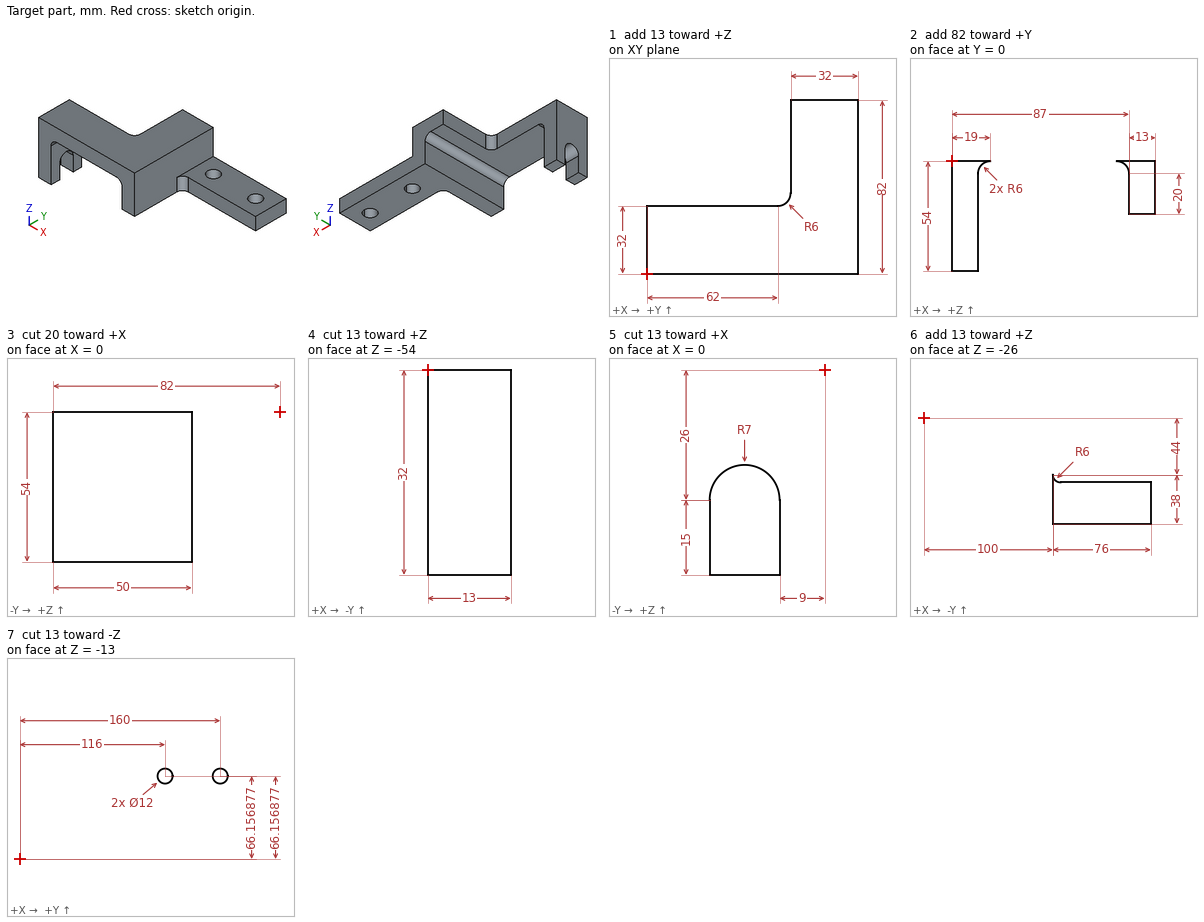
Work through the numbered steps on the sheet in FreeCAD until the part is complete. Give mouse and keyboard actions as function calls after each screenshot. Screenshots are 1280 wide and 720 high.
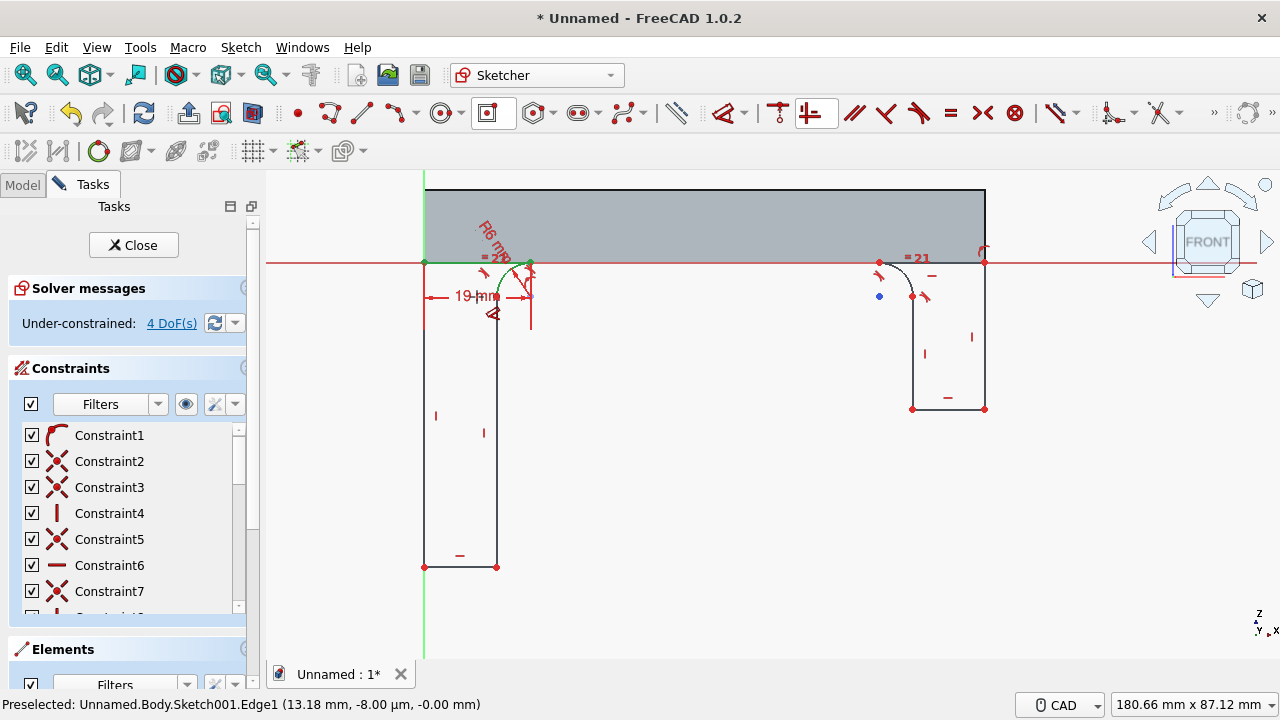
click(424, 354)
click(390, 415)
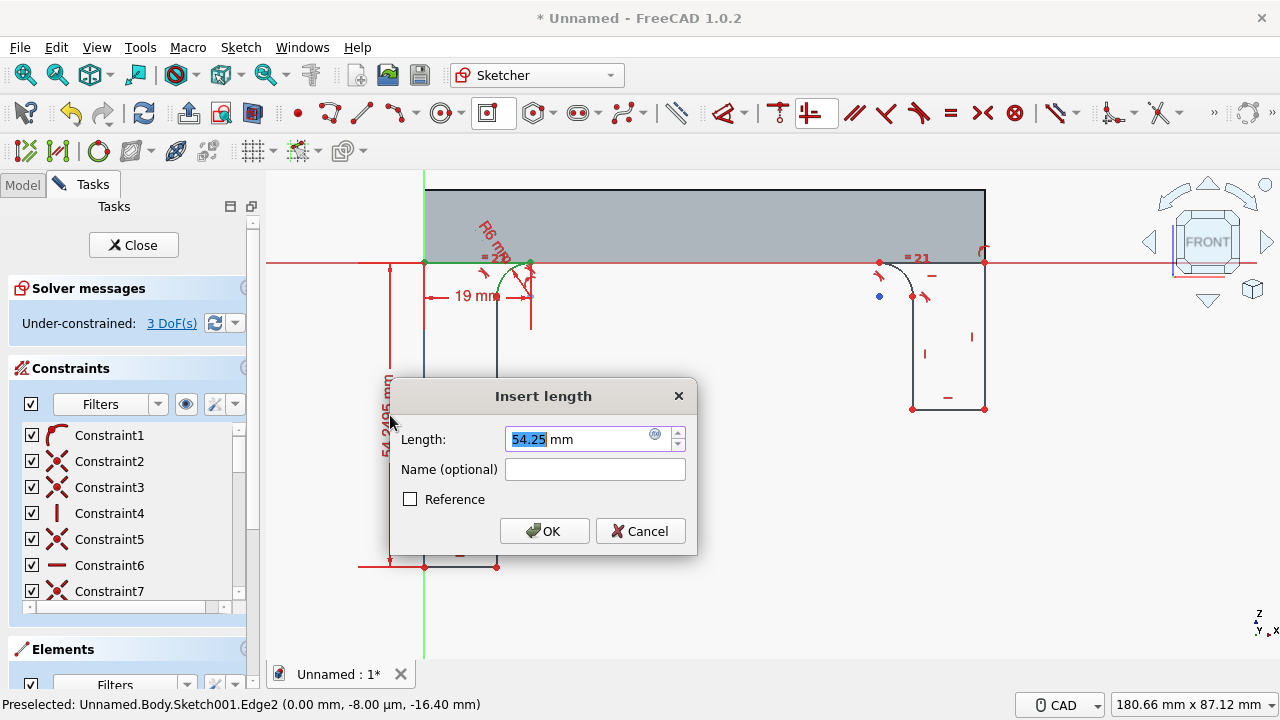
text(54)
key(Return)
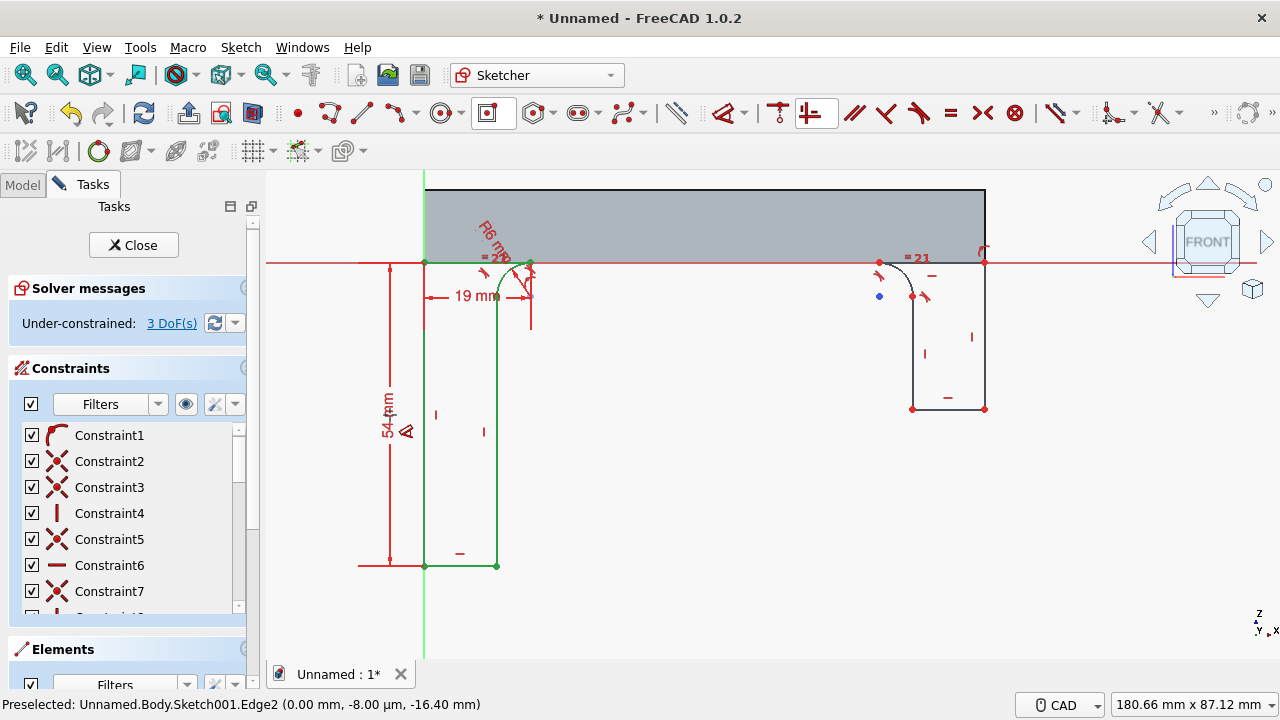
click(913, 331)
click(947, 353)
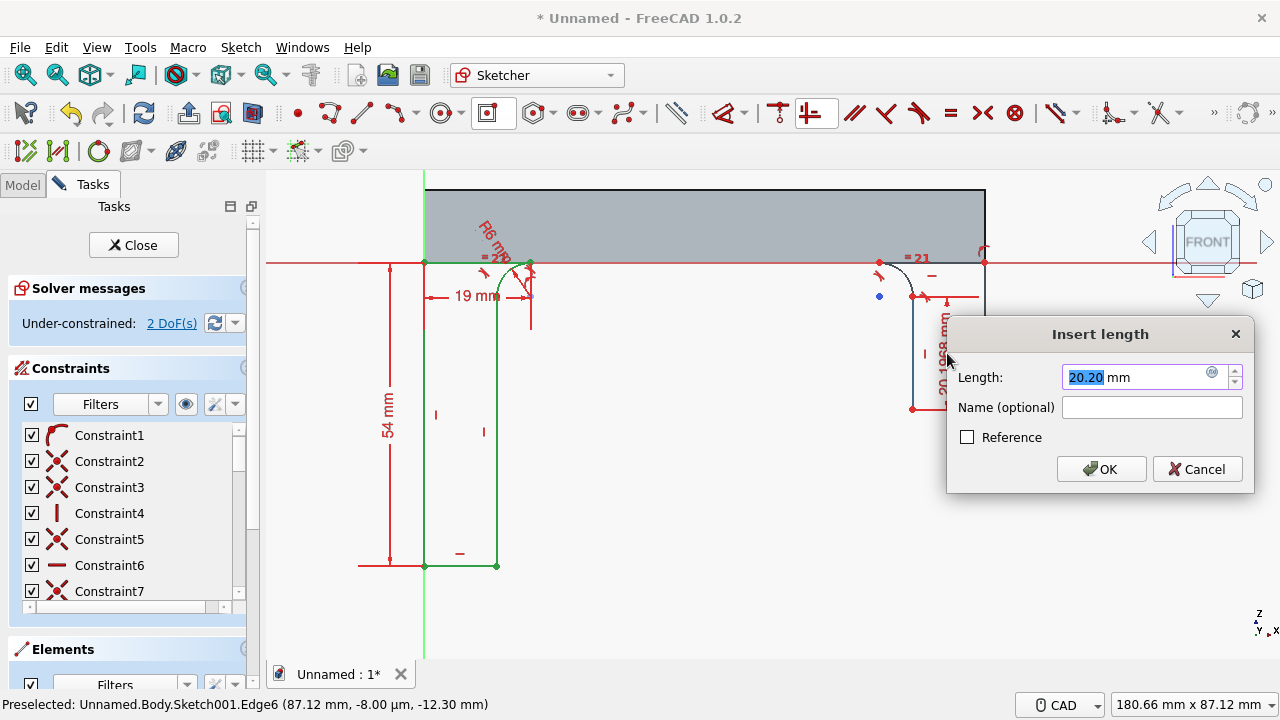
text(20)
key(Return)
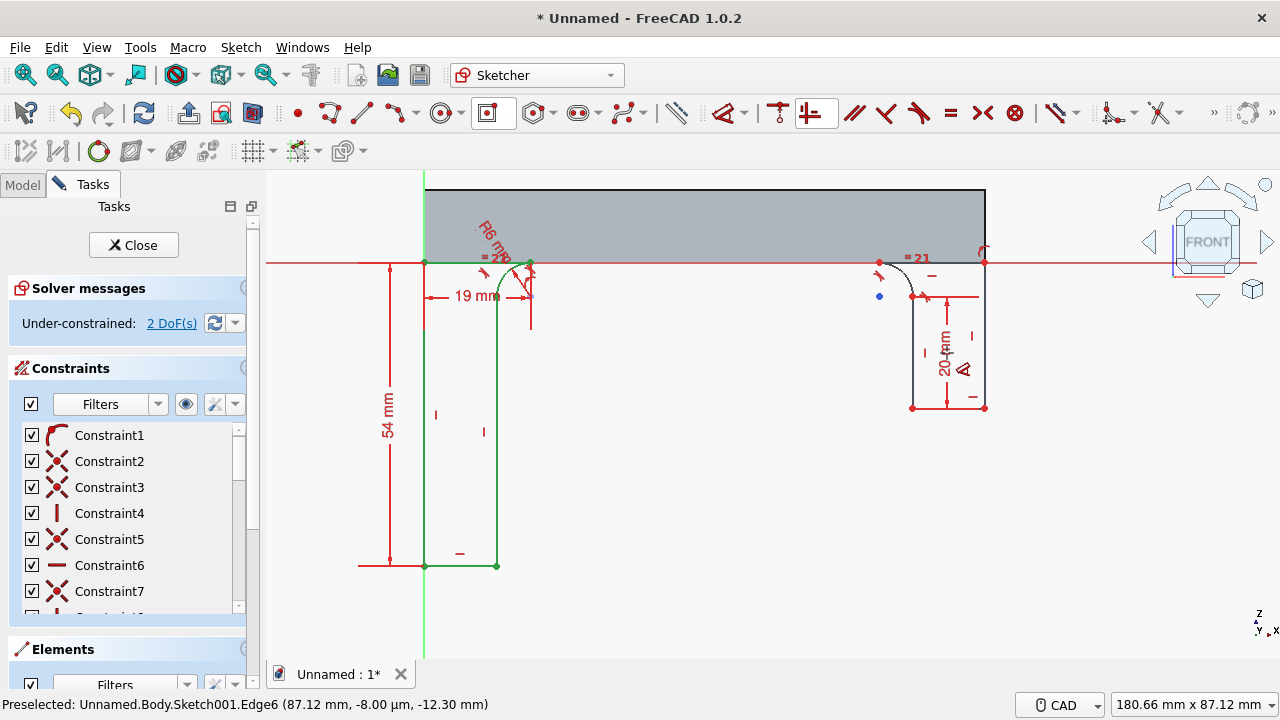
click(935, 409)
click(949, 375)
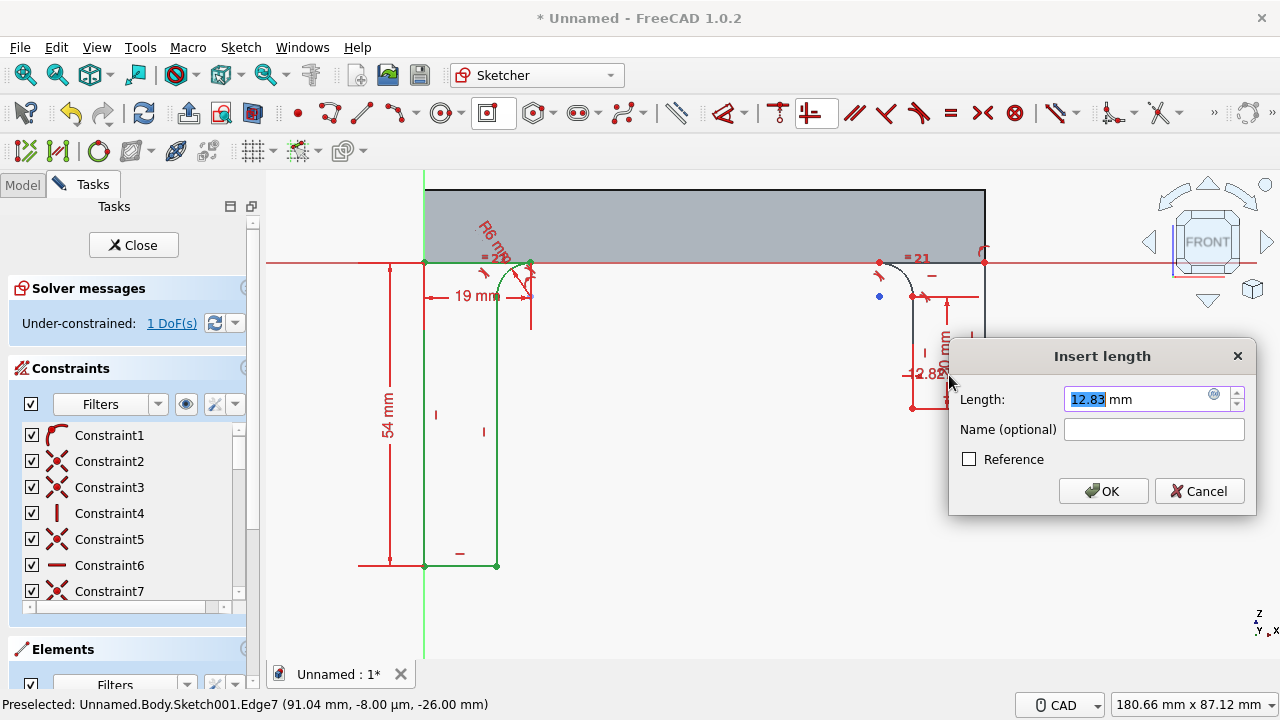
text(13)
key(Return)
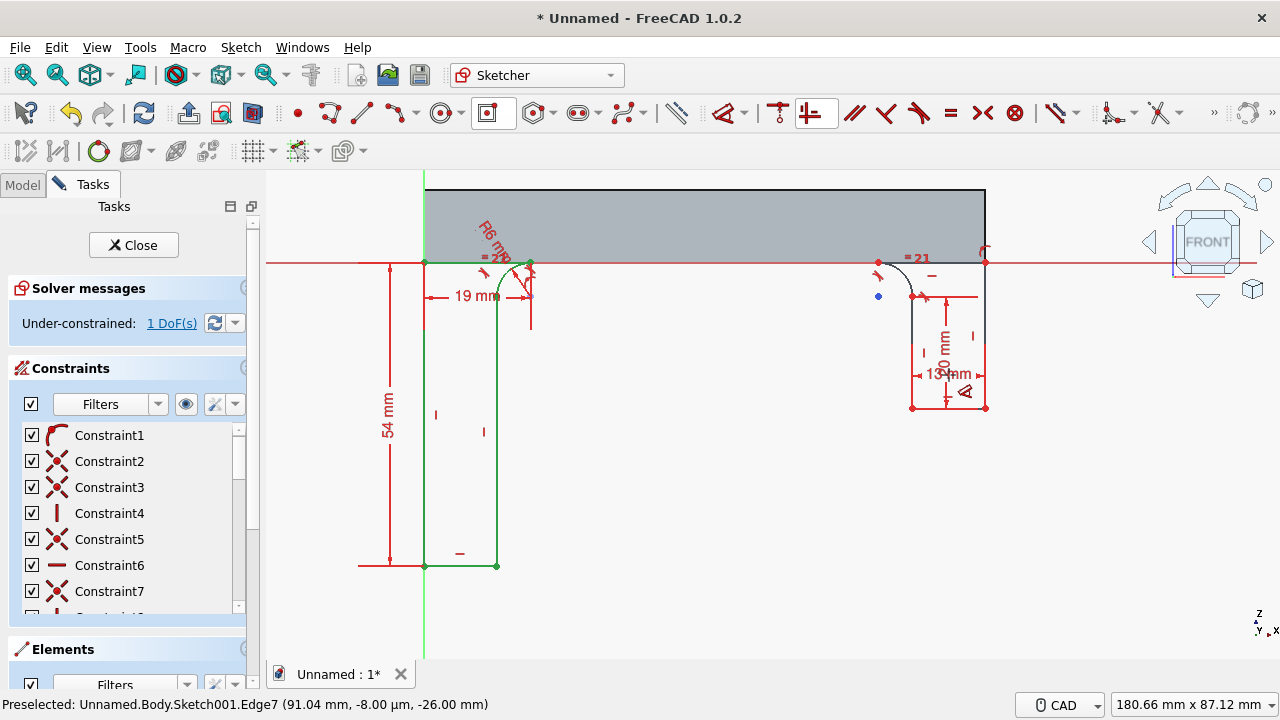
click(912, 297)
click(668, 229)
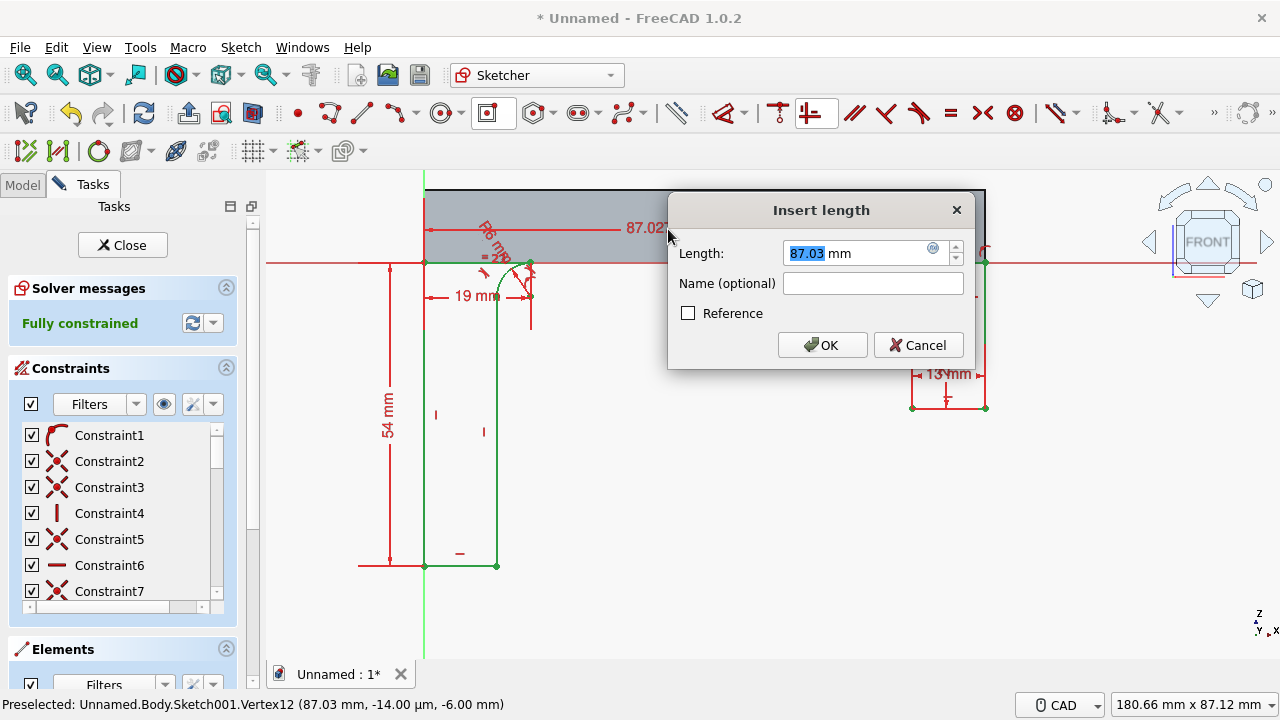
text(87)
key(Return)
key(Escape)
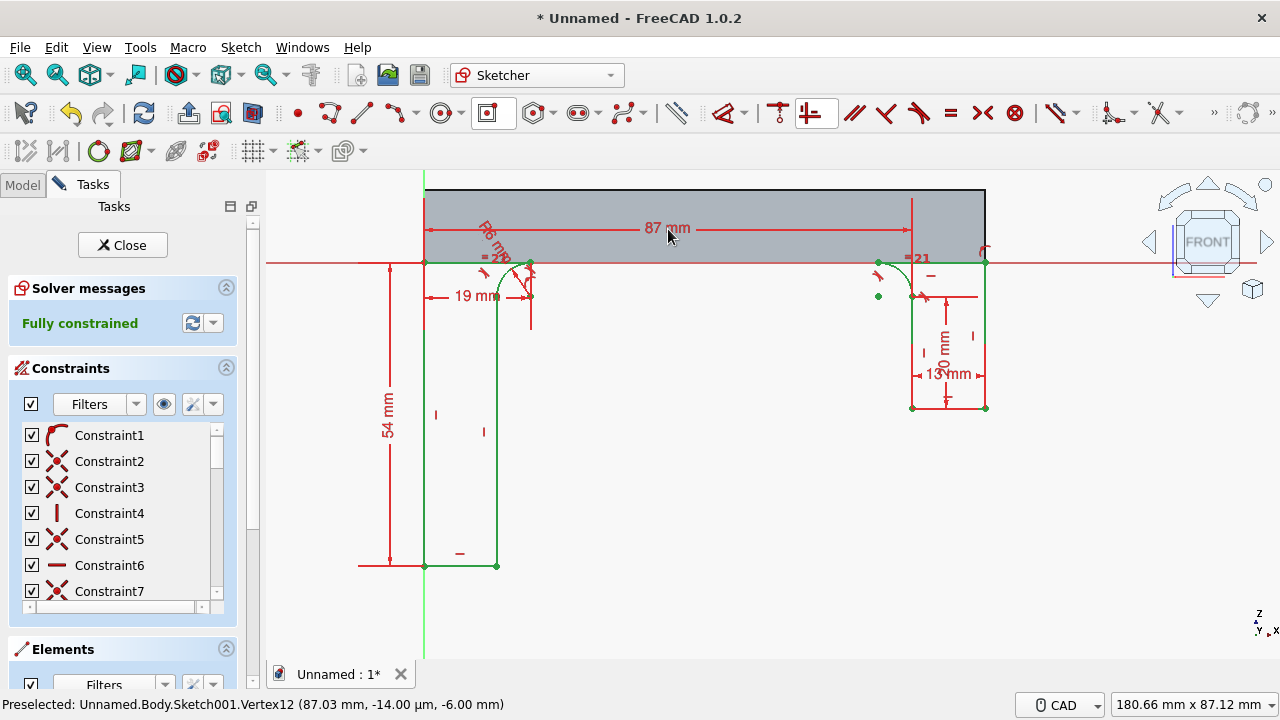
click(123, 245)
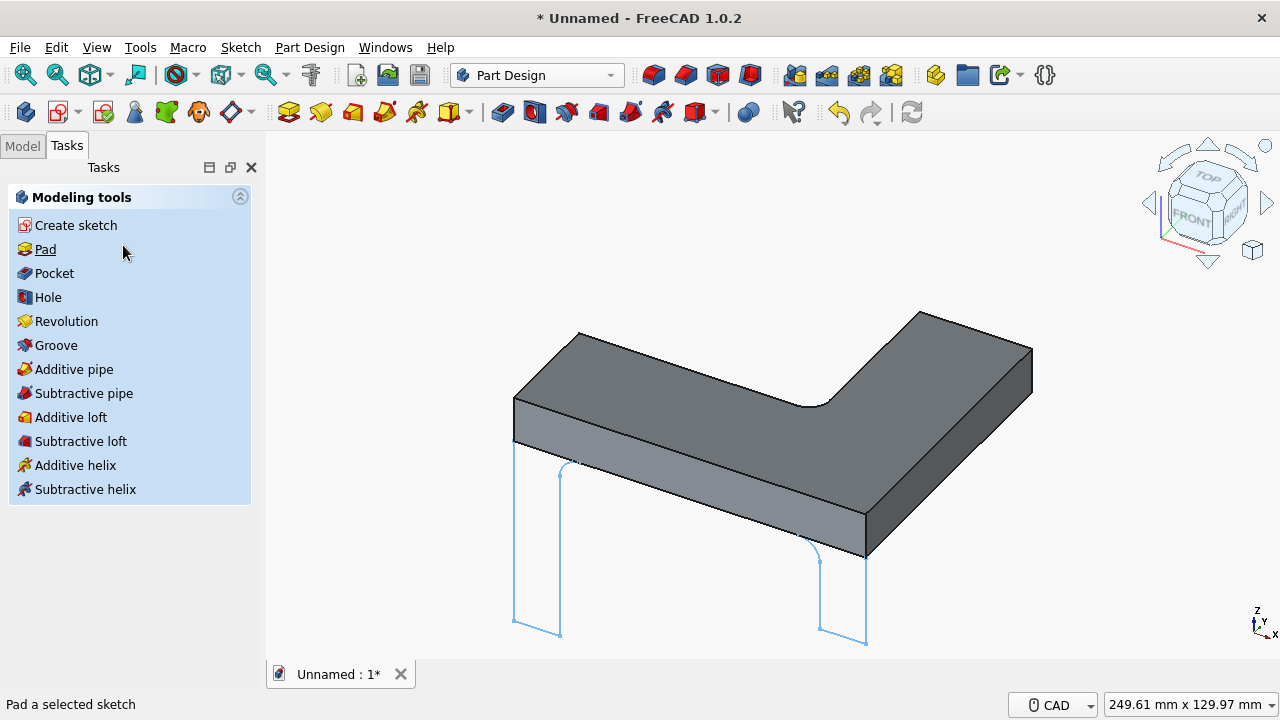
click(290, 112)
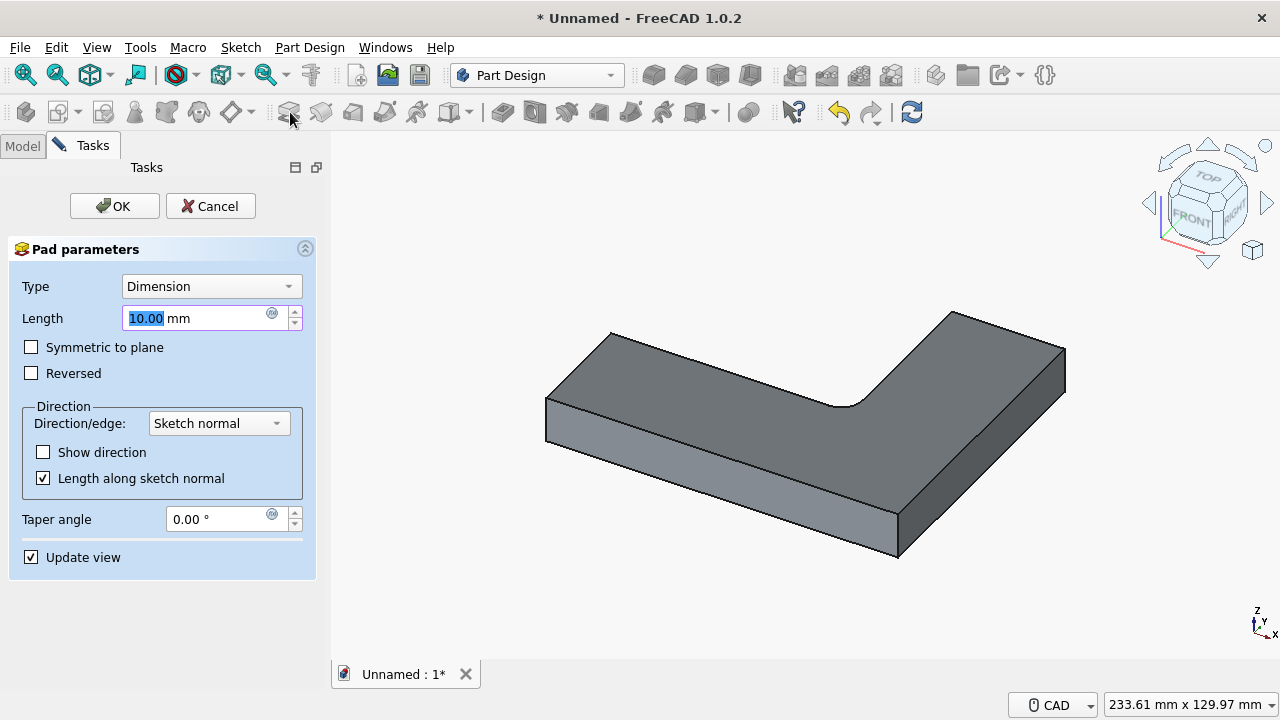
text(82)
key(Tab)